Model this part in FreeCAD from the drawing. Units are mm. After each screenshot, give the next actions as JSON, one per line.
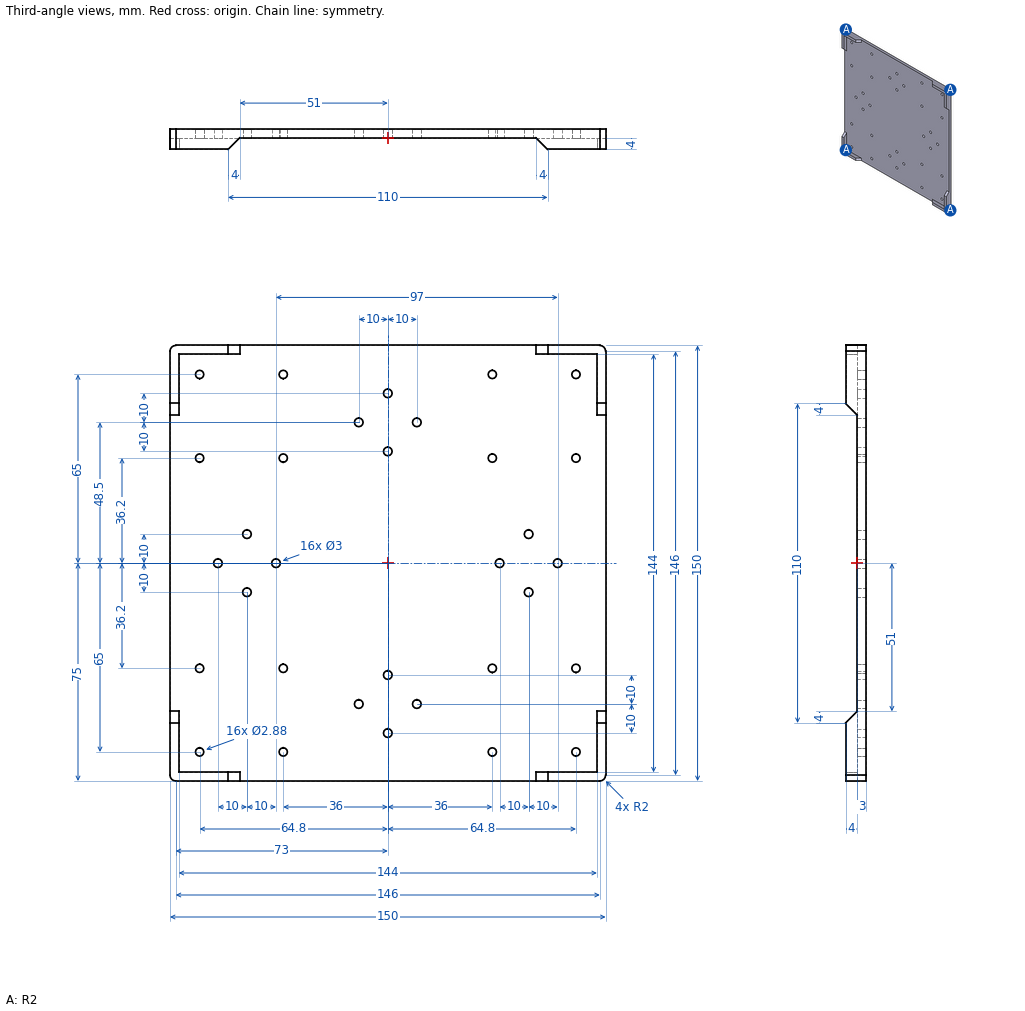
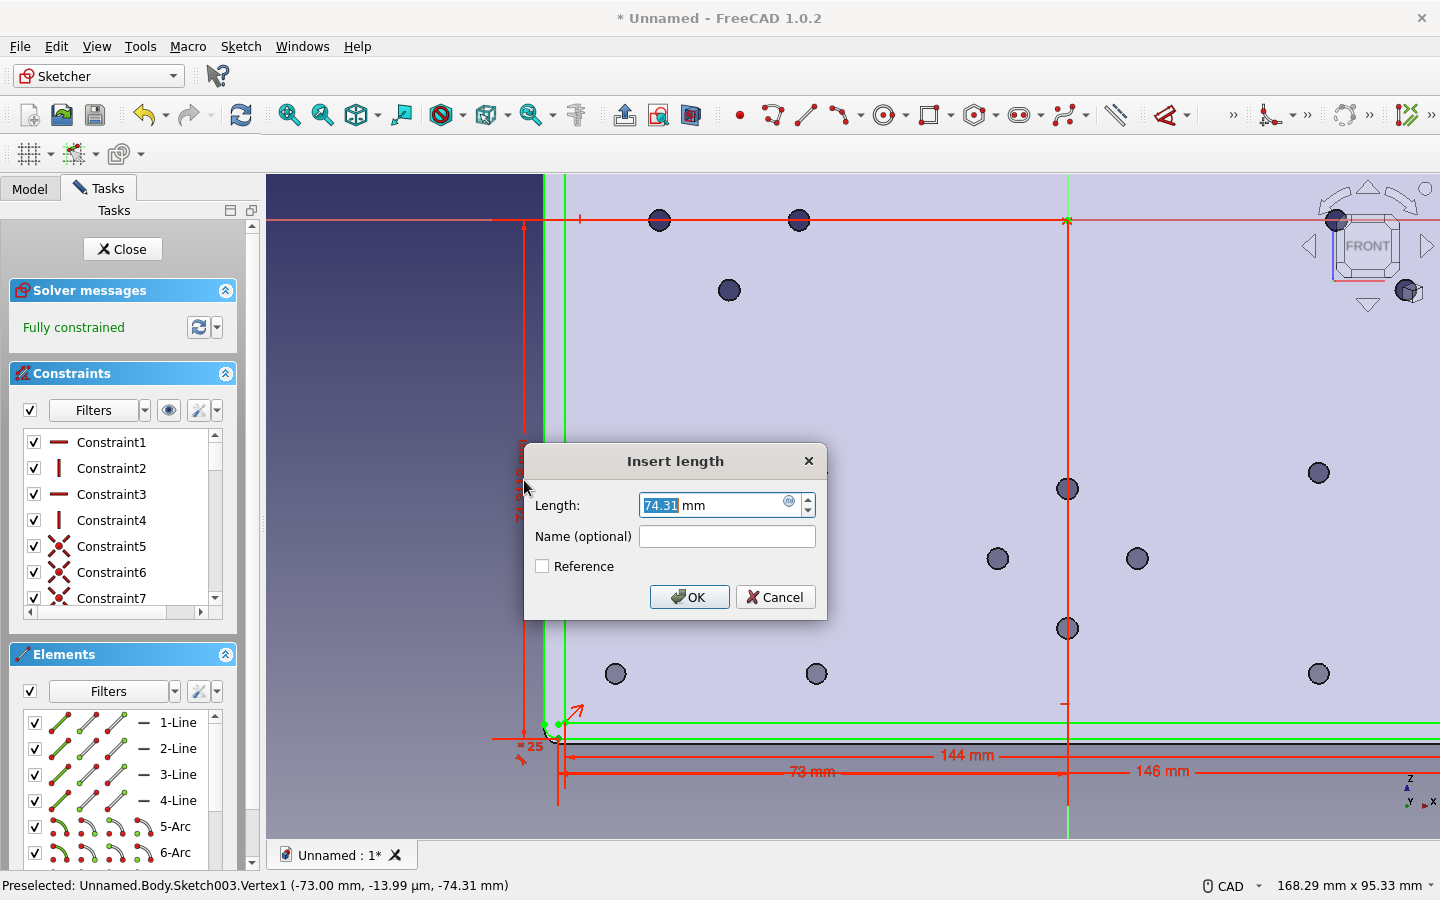
{"action": "type", "text": "75"}
{"action": "key", "text": "Return"}
{"action": "key", "text": "Escape"}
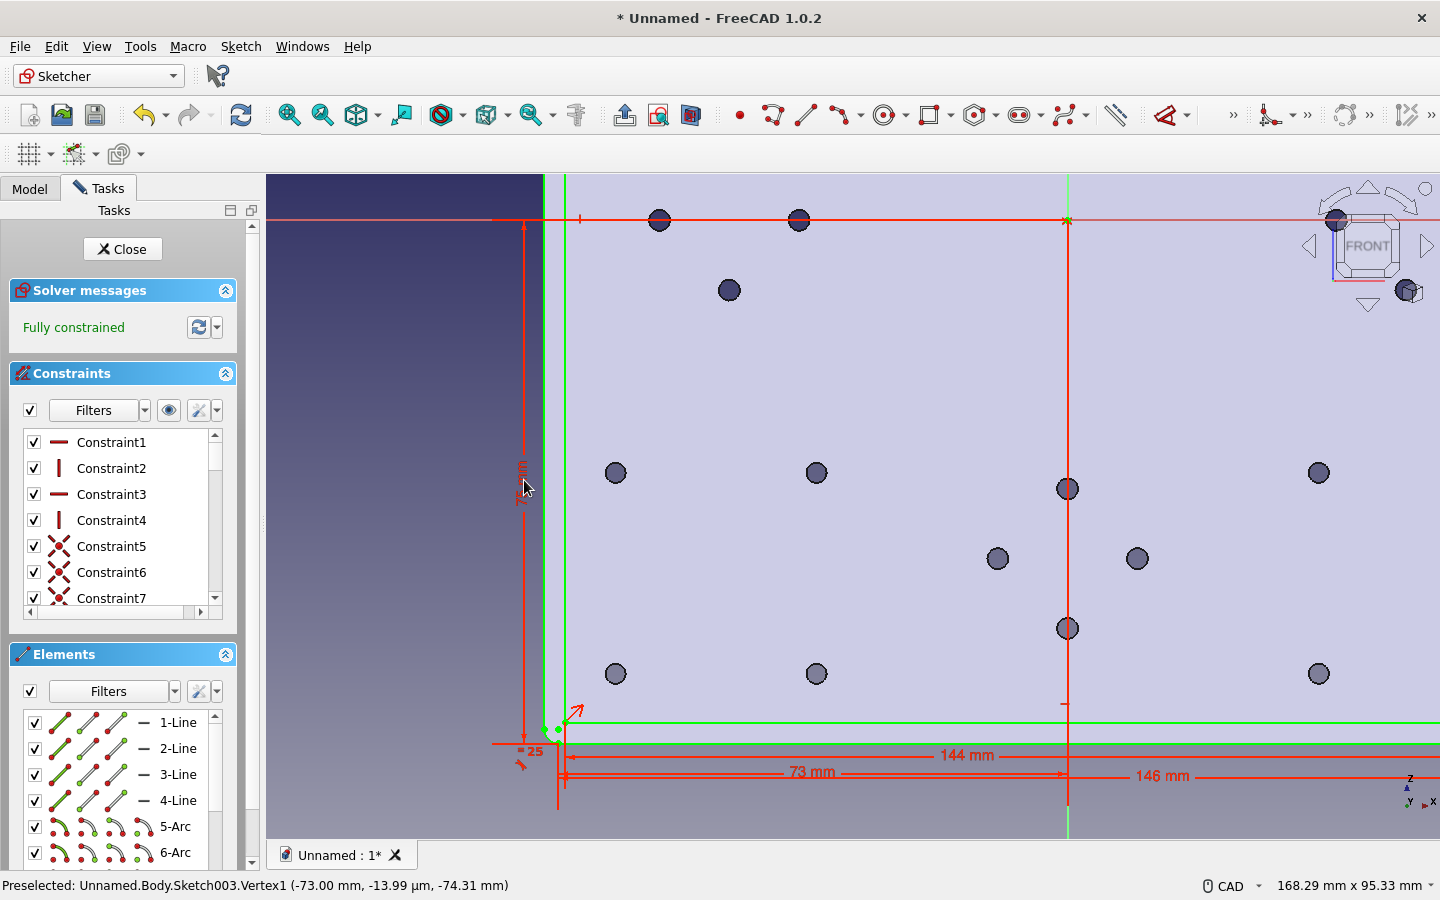
{"action": "left_click", "coordinate": [123, 249]}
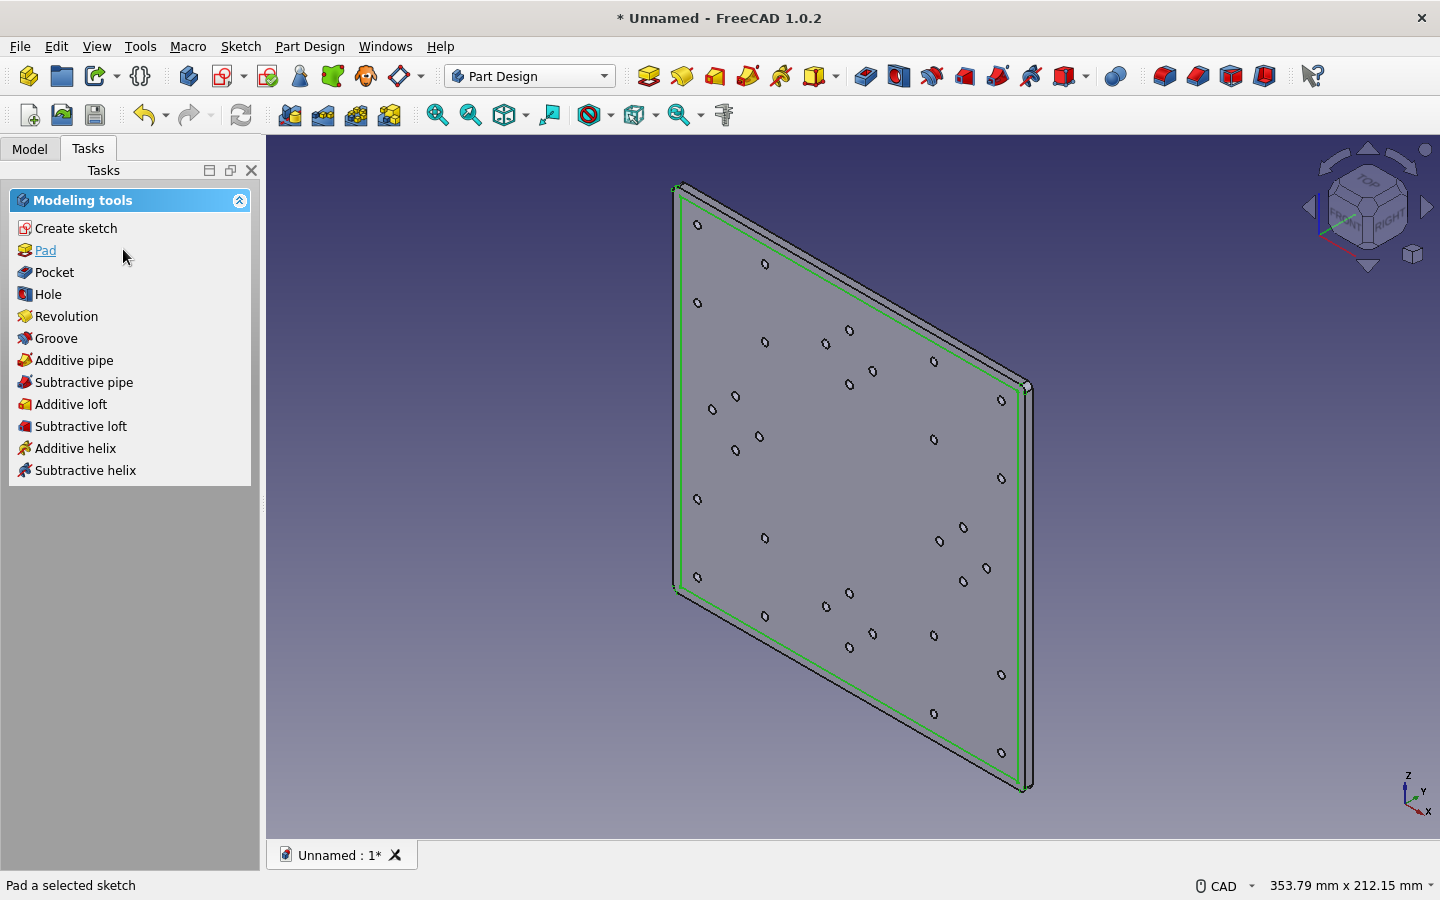
{"action": "left_click", "coordinate": [649, 76]}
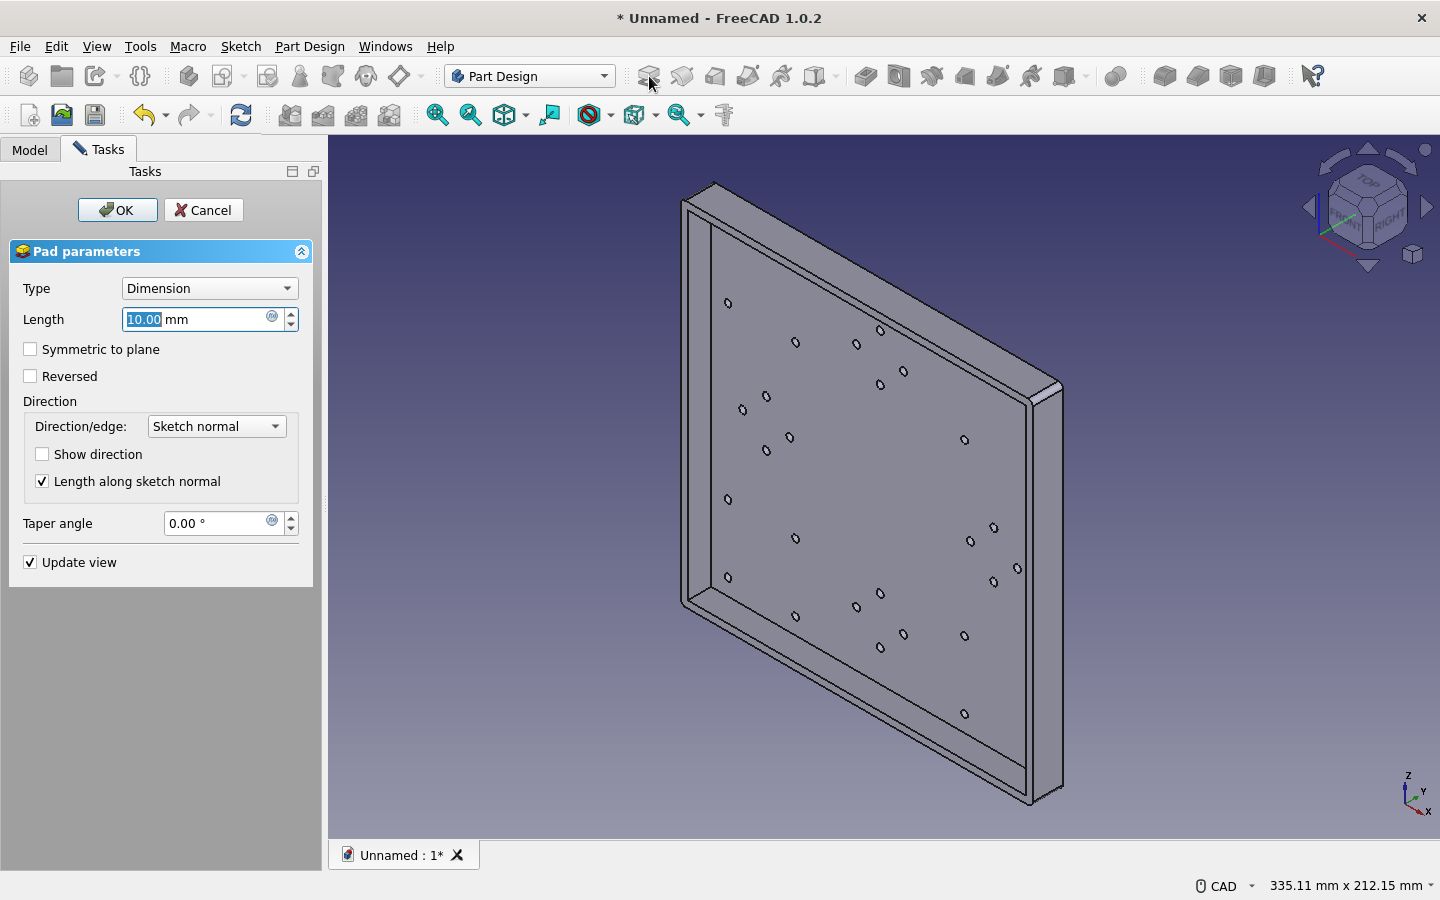
{"action": "type", "text": "4"}
{"action": "key", "text": "Tab"}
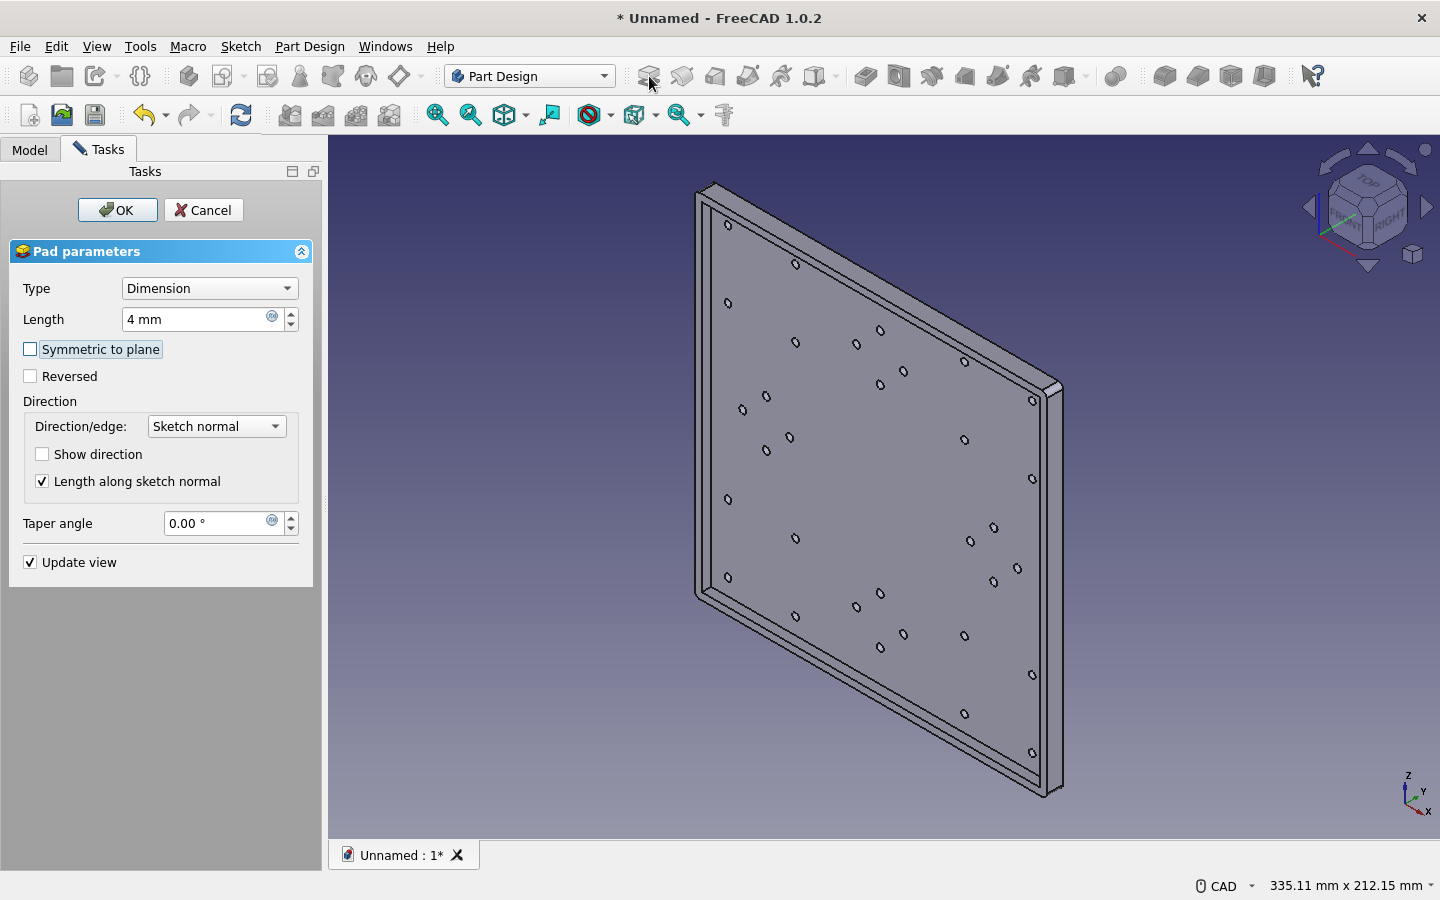
{"action": "left_click", "coordinate": [118, 210]}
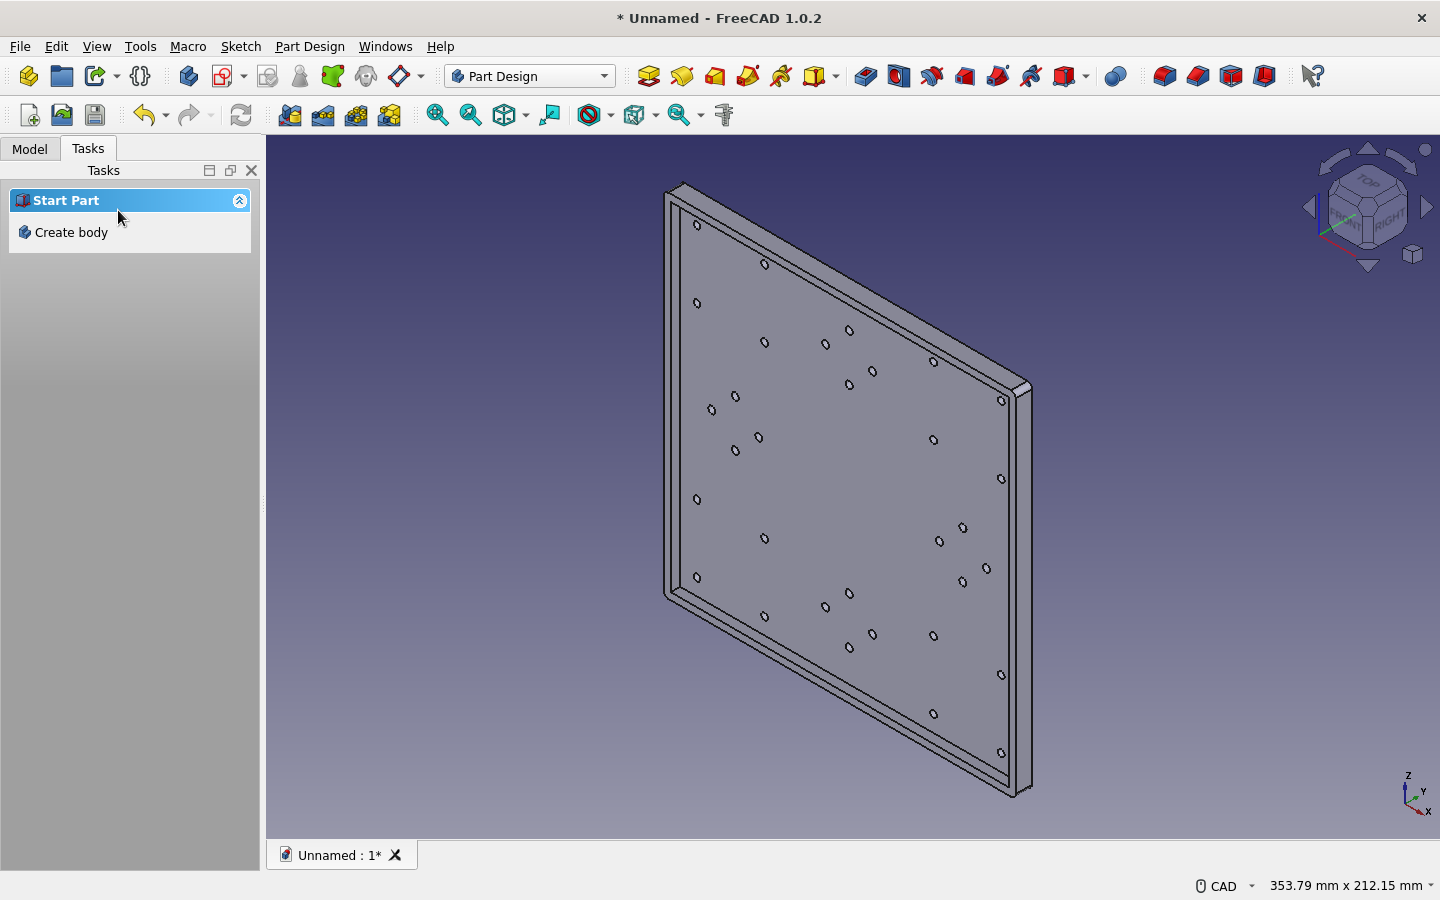
{"action": "left_click", "coordinate": [997, 369]}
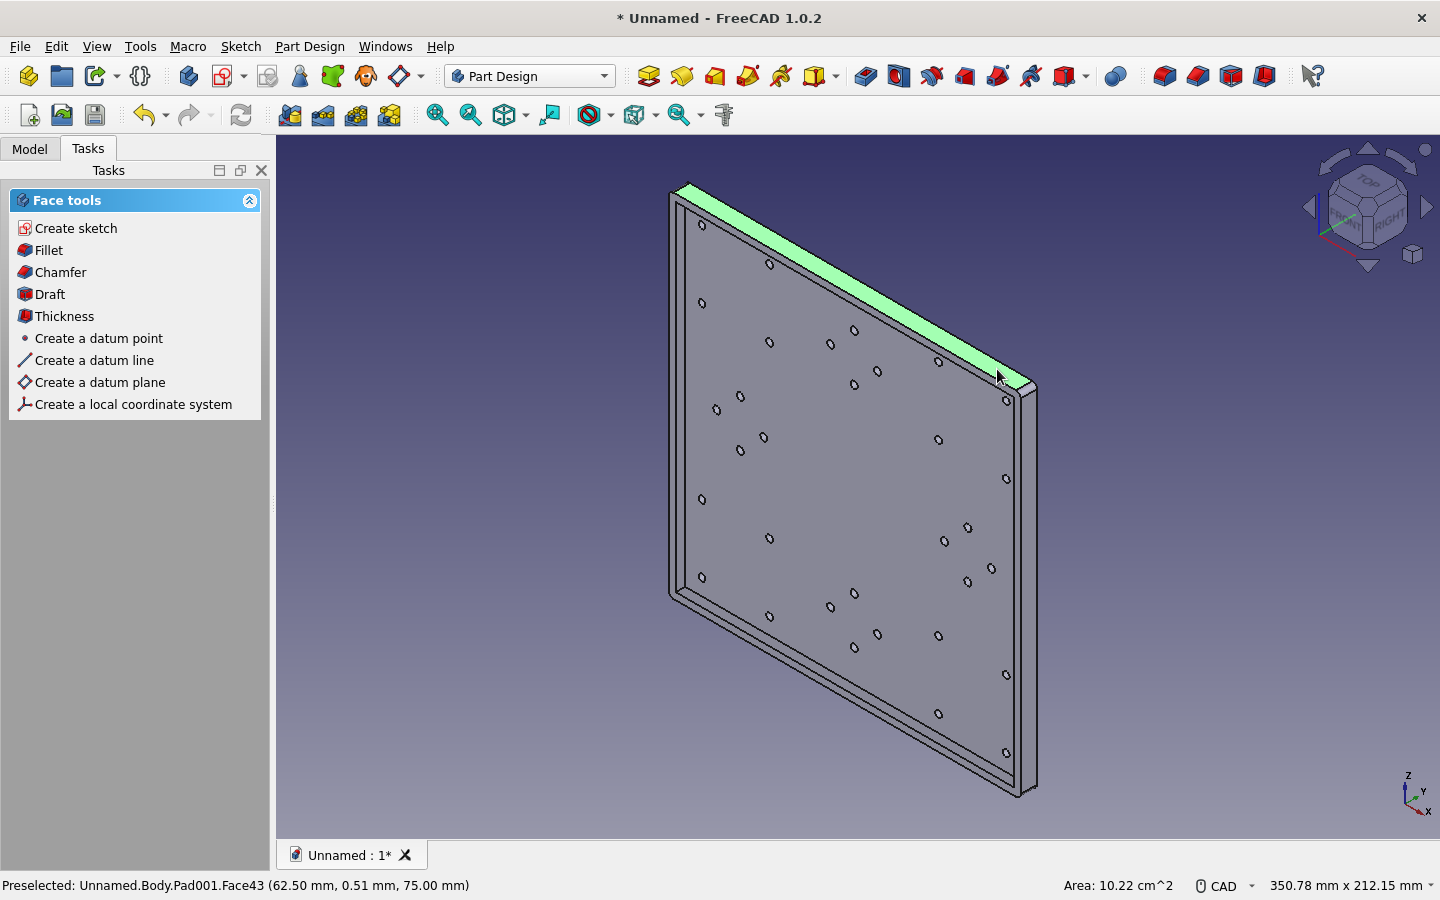
{"action": "left_click", "coordinate": [222, 76]}